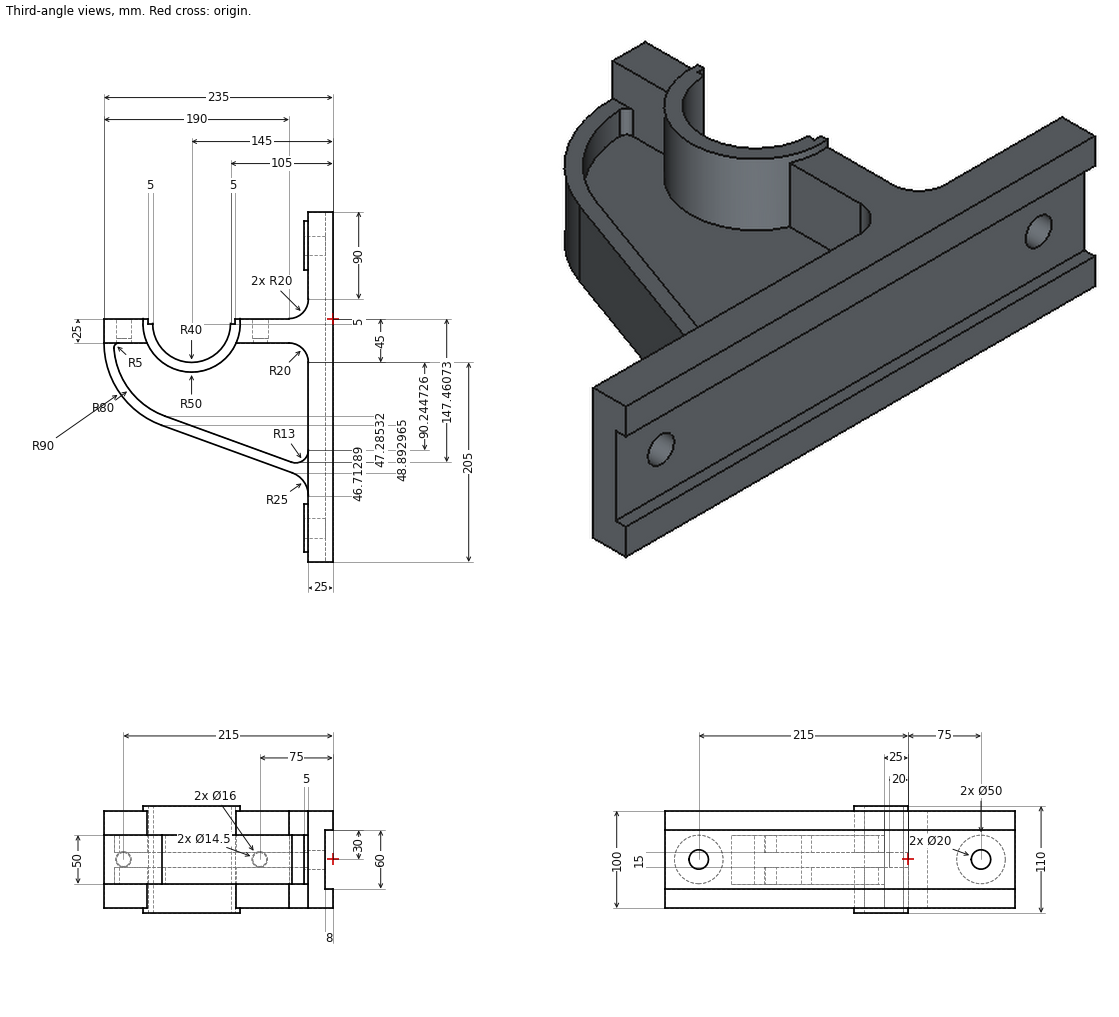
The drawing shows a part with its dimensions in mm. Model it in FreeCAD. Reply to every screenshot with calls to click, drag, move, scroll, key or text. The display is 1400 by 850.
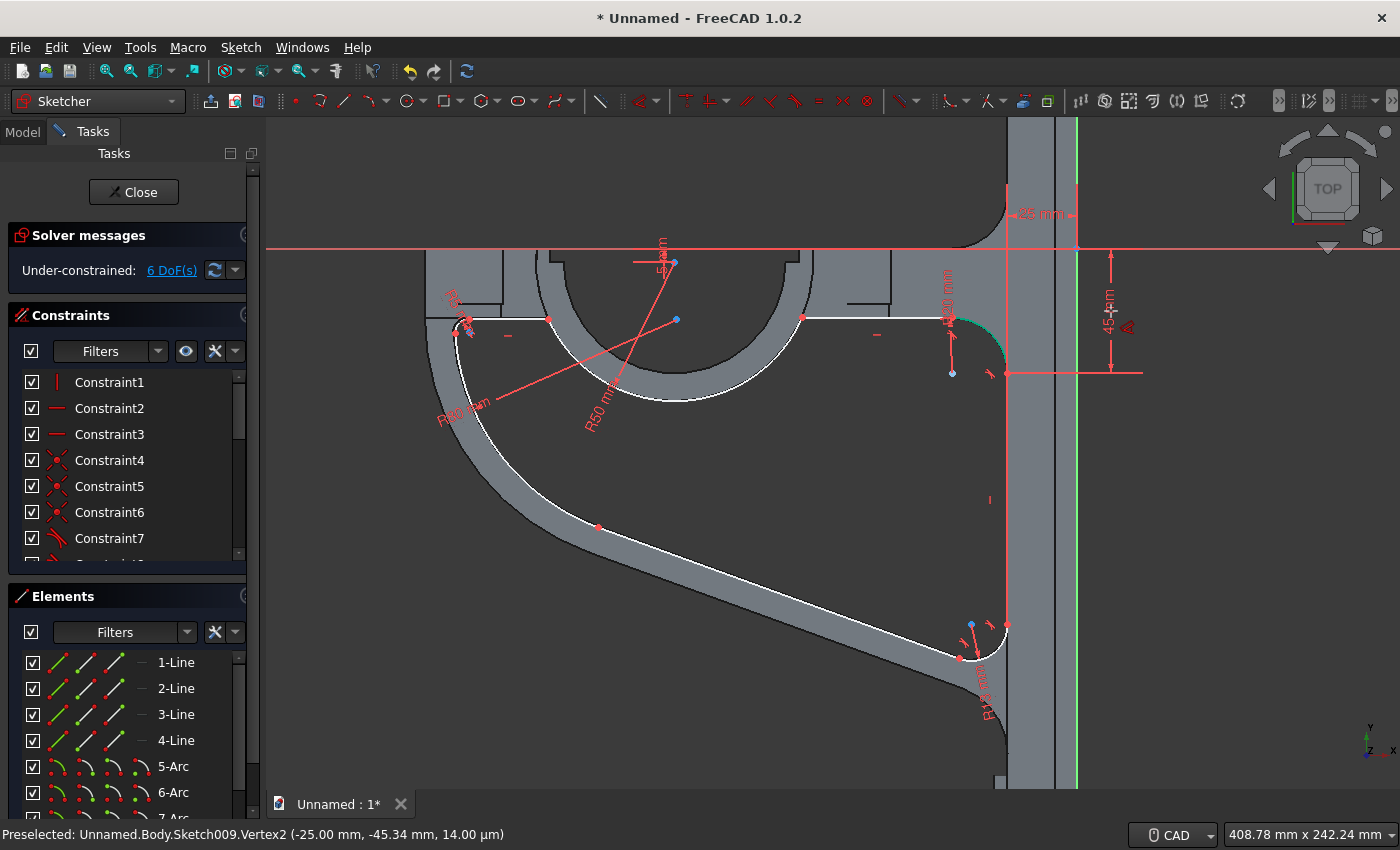
click(548, 319)
click(1111, 284)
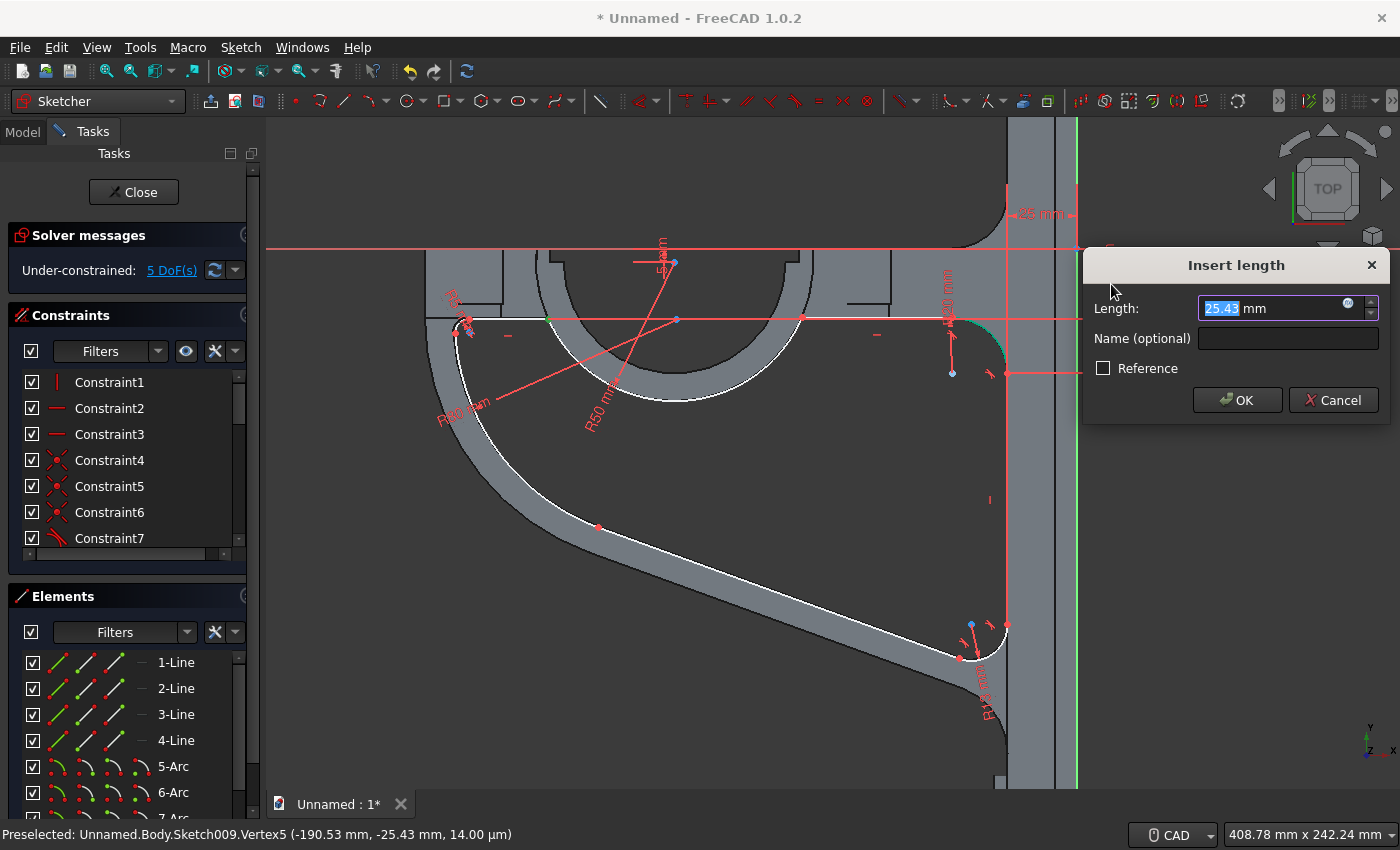
text(25)
key(Return)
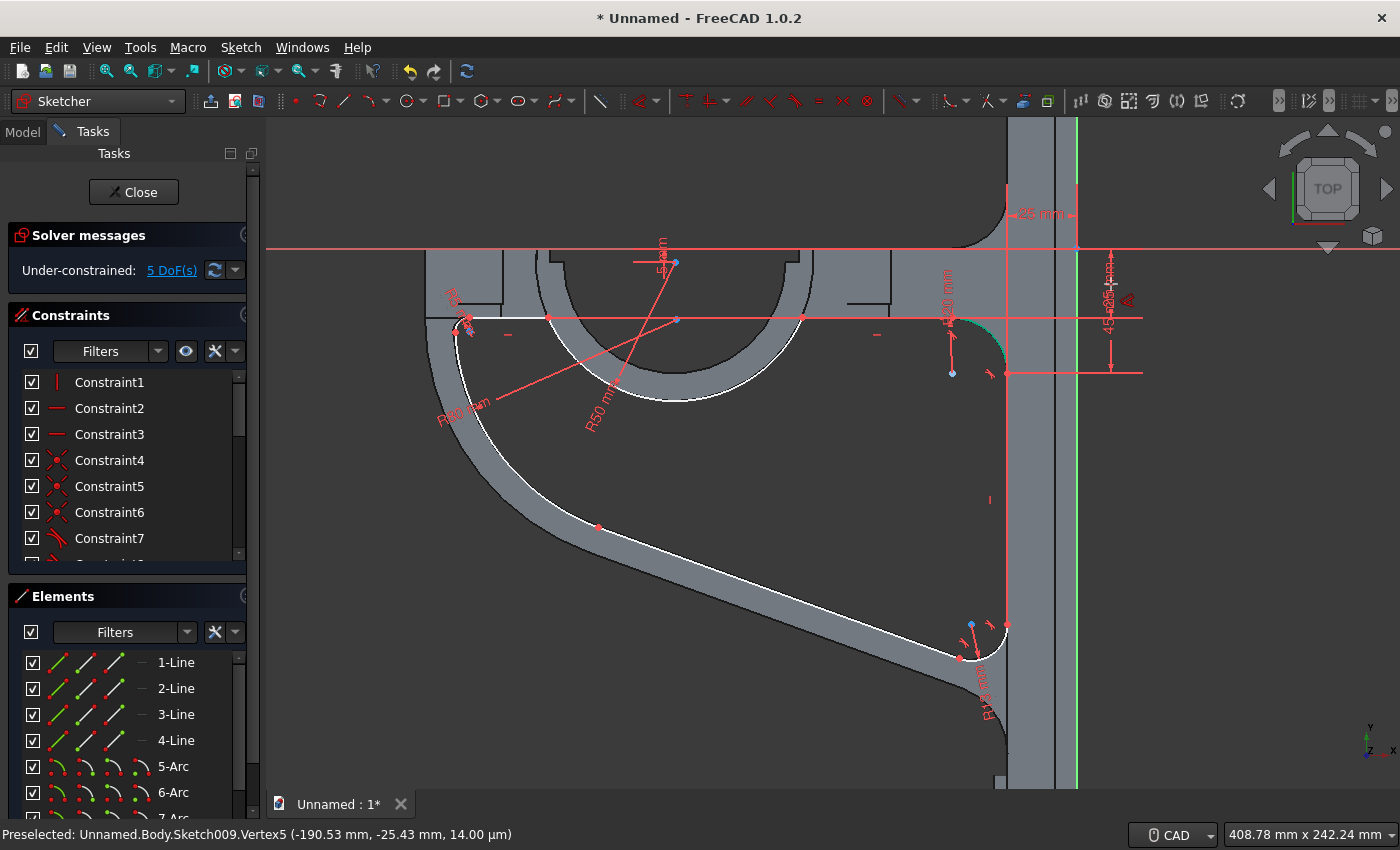
click(677, 320)
click(643, 284)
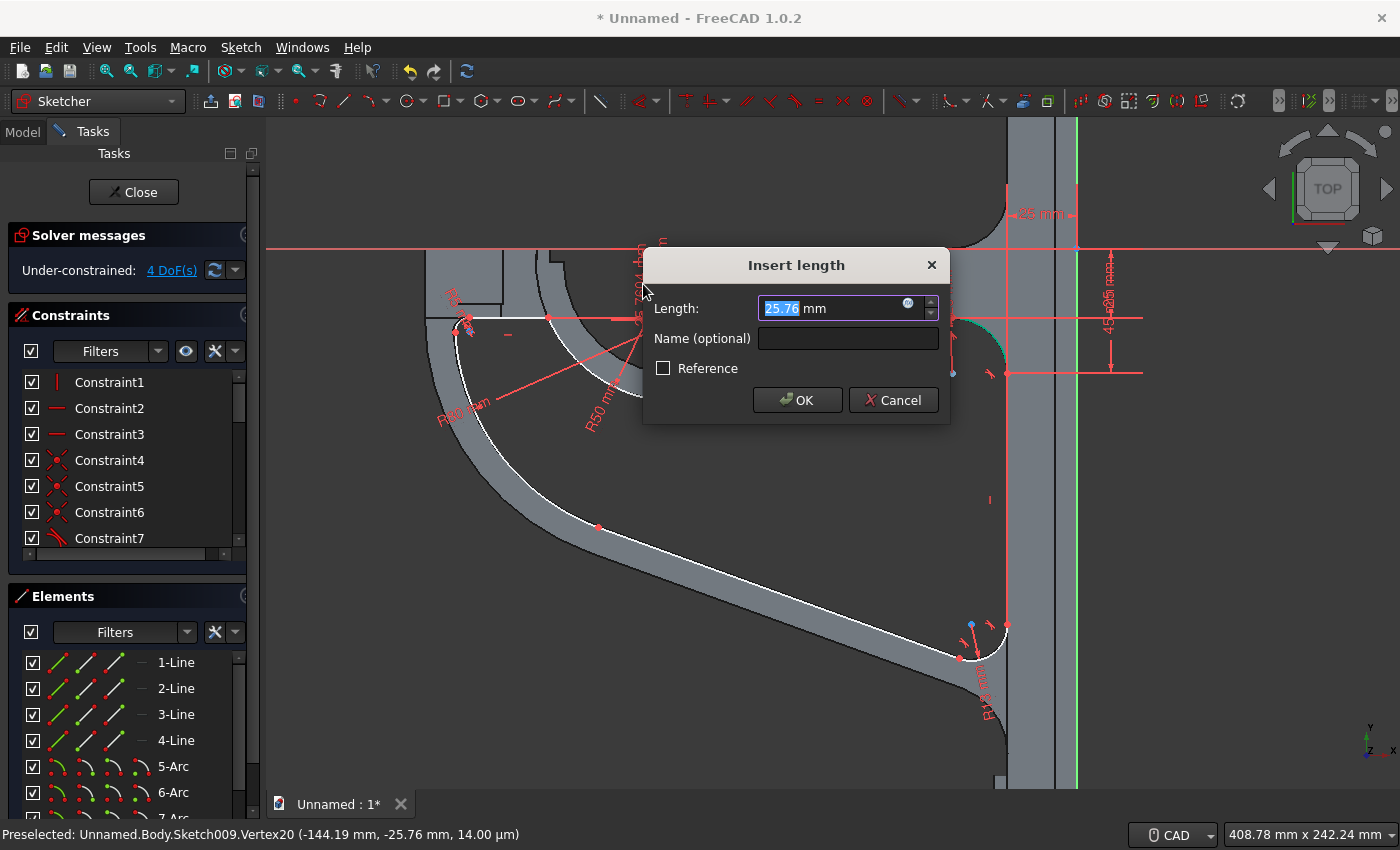
text(25)
key(Return)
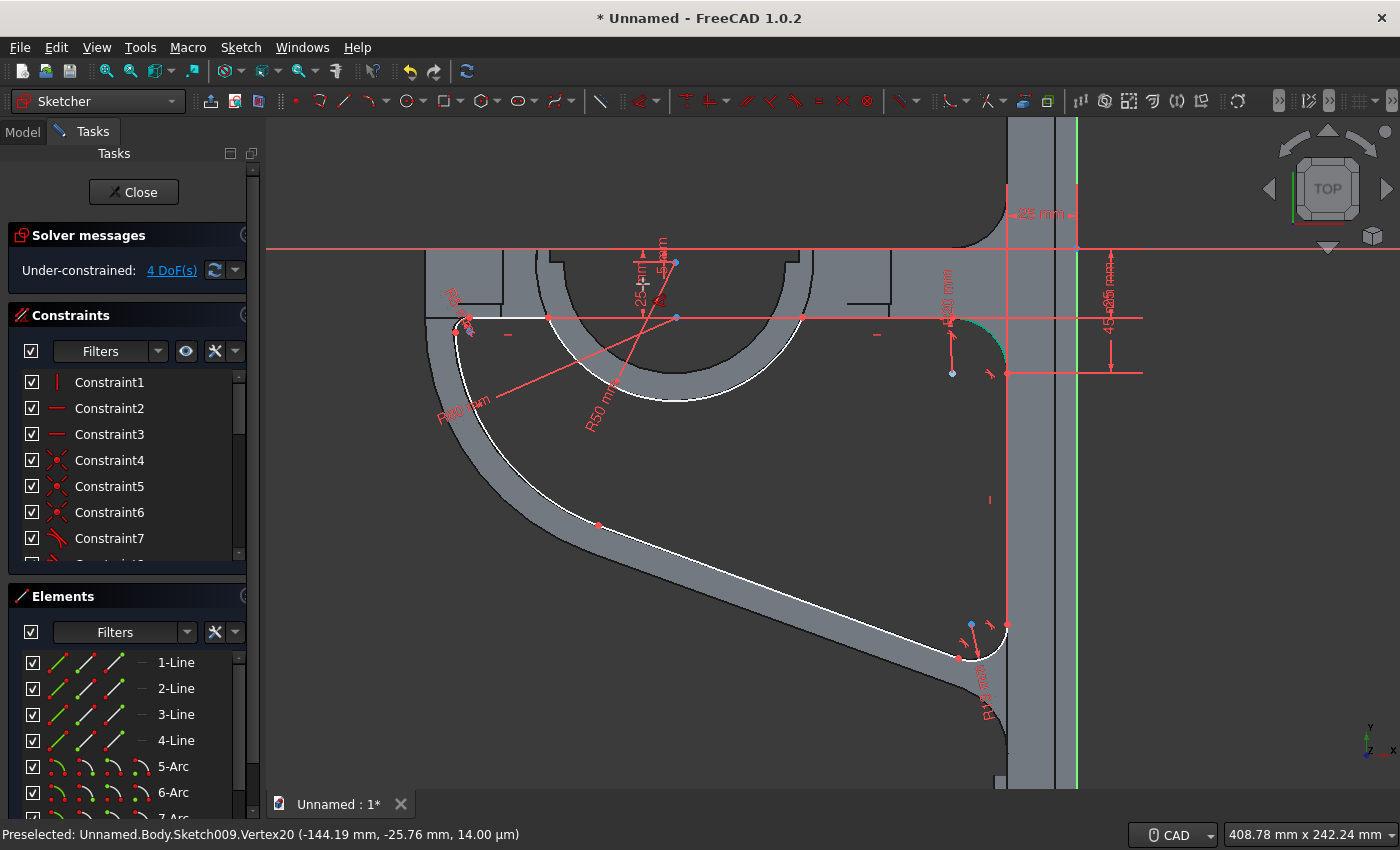
click(675, 262)
click(876, 215)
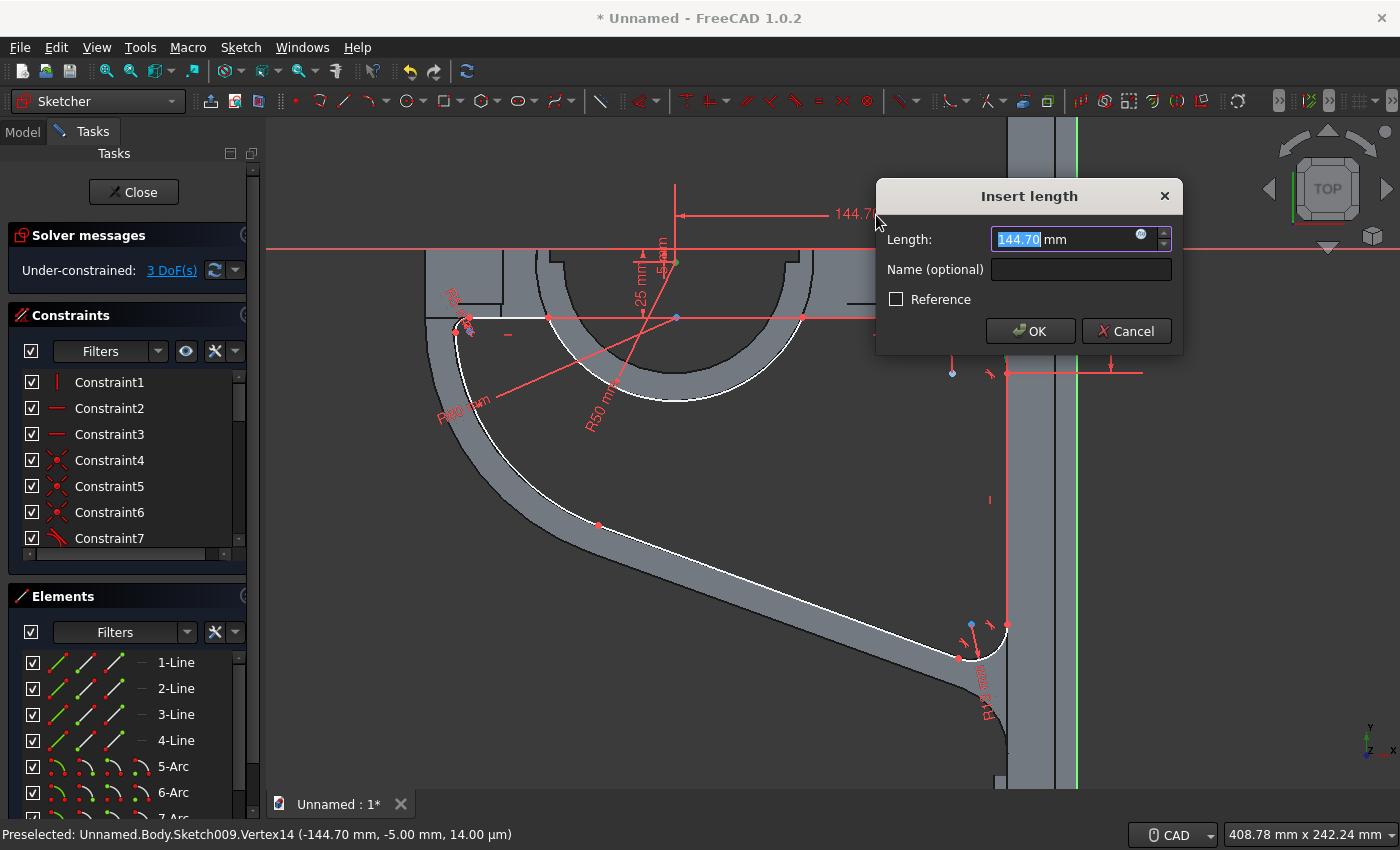
text(145)
key(Return)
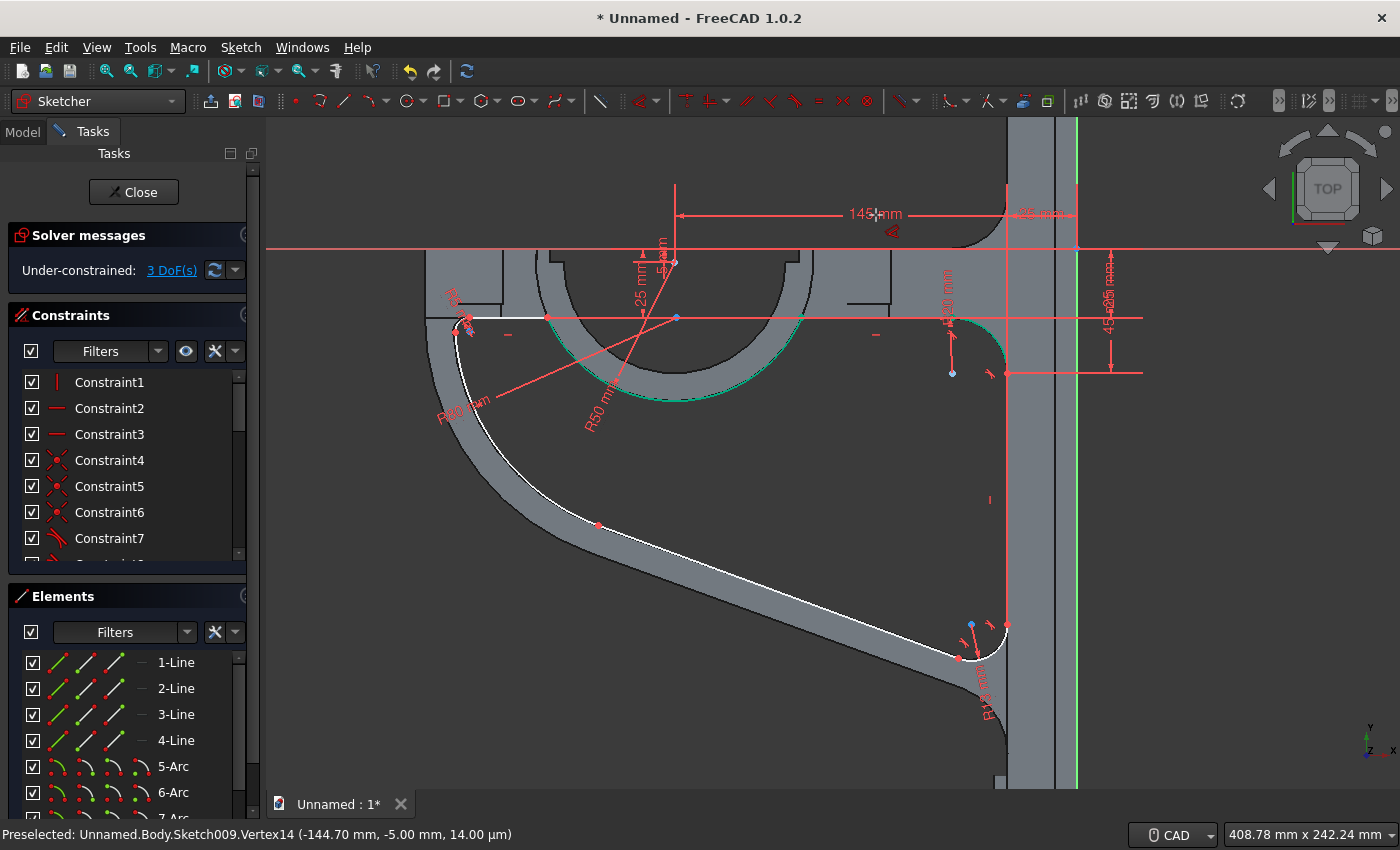
click(677, 318)
click(785, 215)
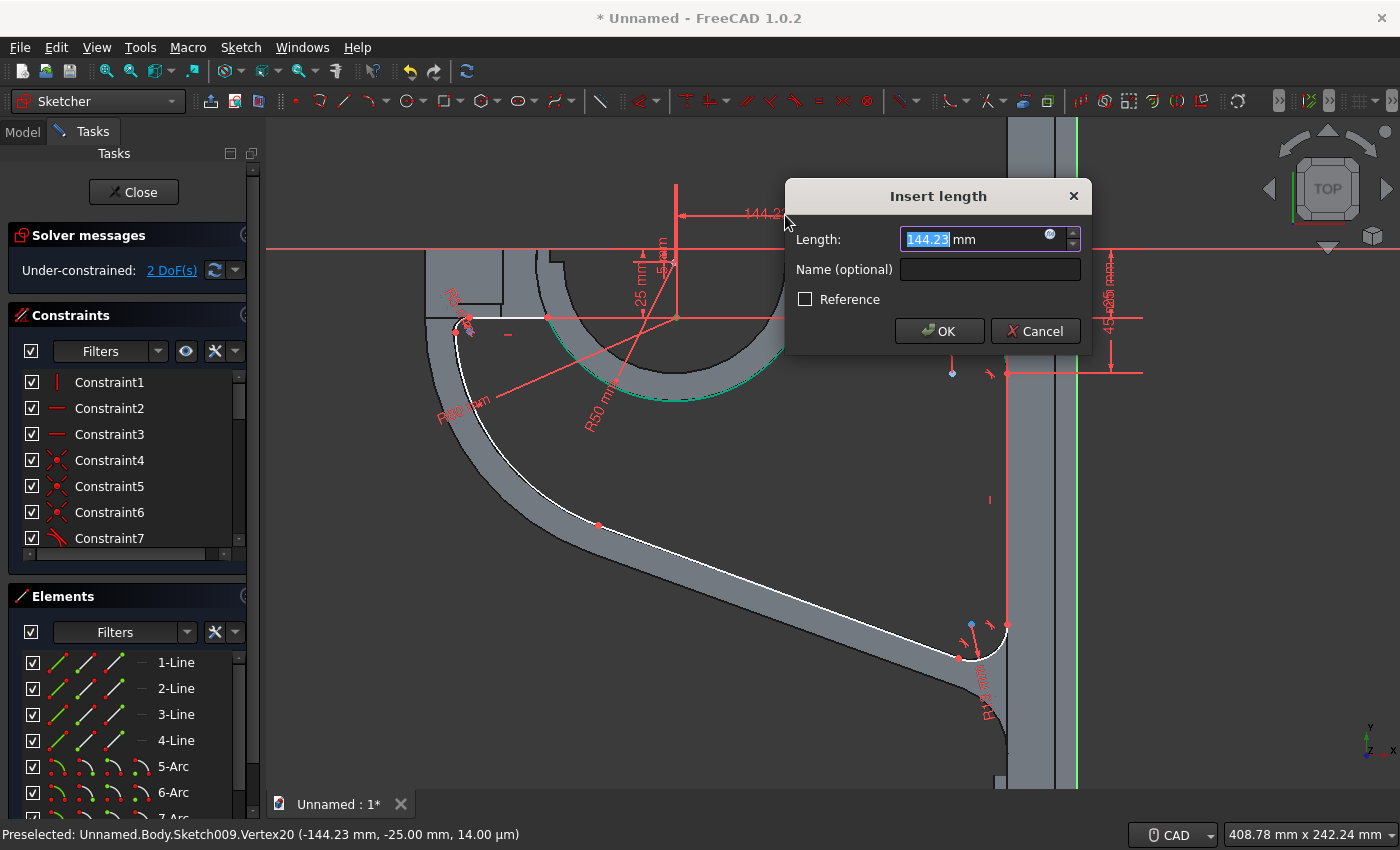
text(145)
key(Return)